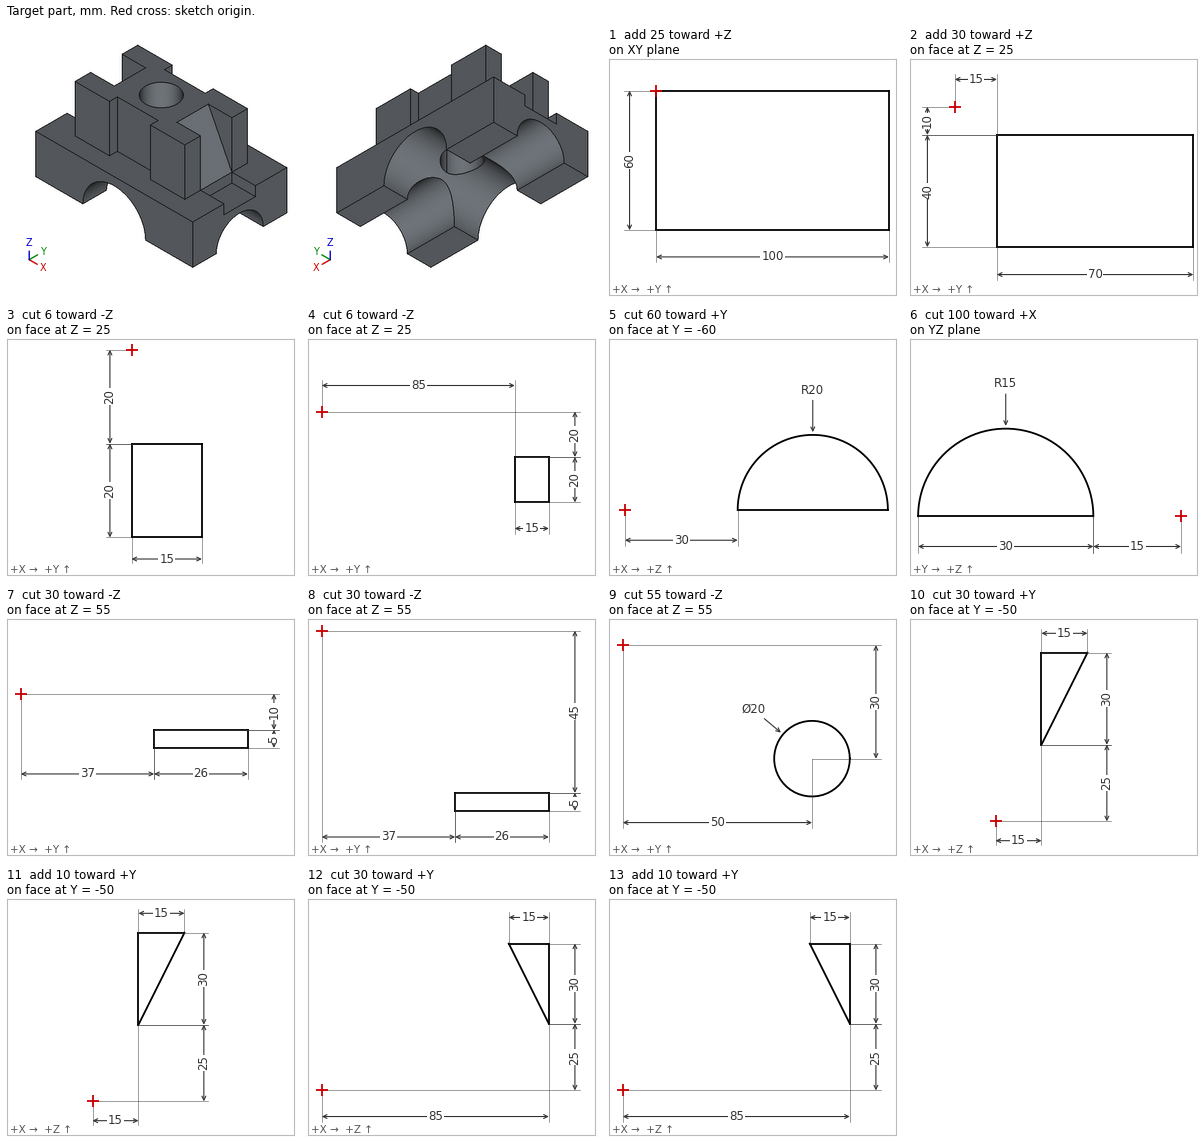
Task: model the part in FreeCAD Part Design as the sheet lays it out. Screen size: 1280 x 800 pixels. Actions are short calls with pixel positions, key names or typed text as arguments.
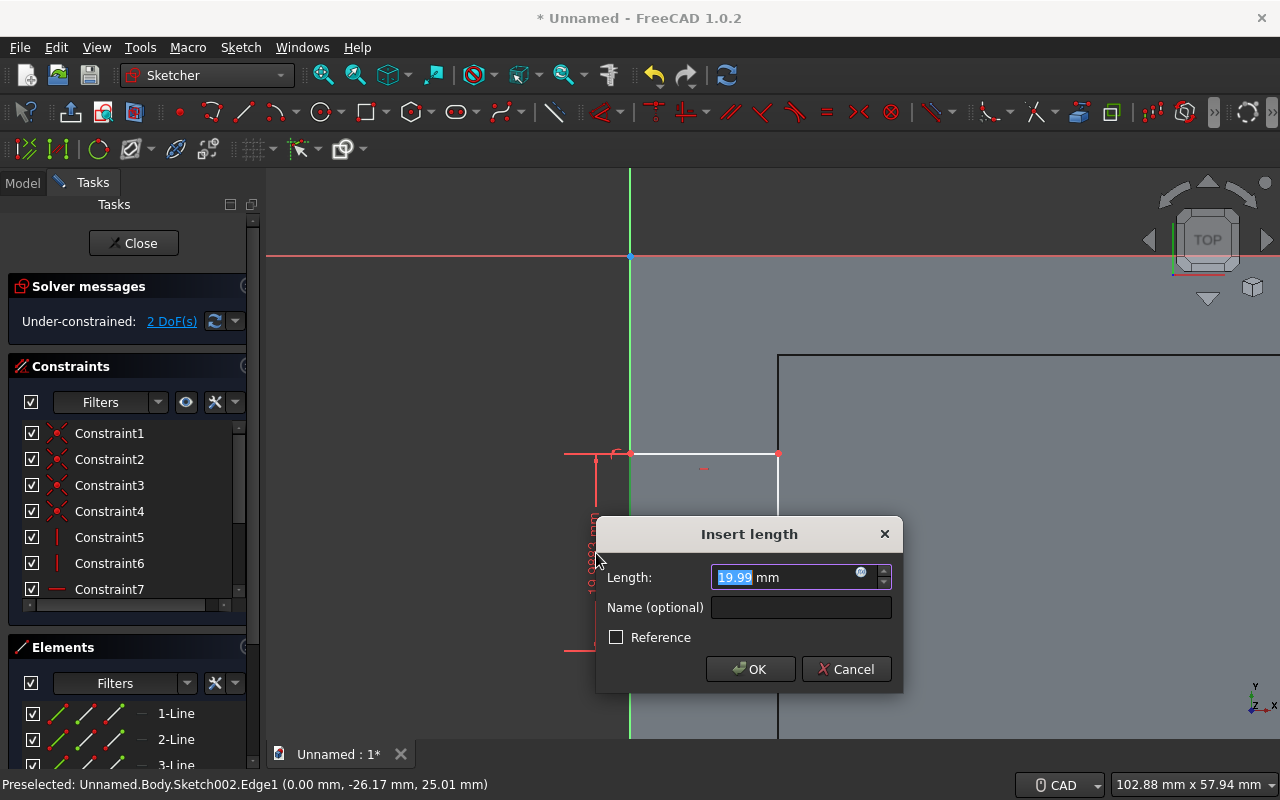
text(20)
key(Return)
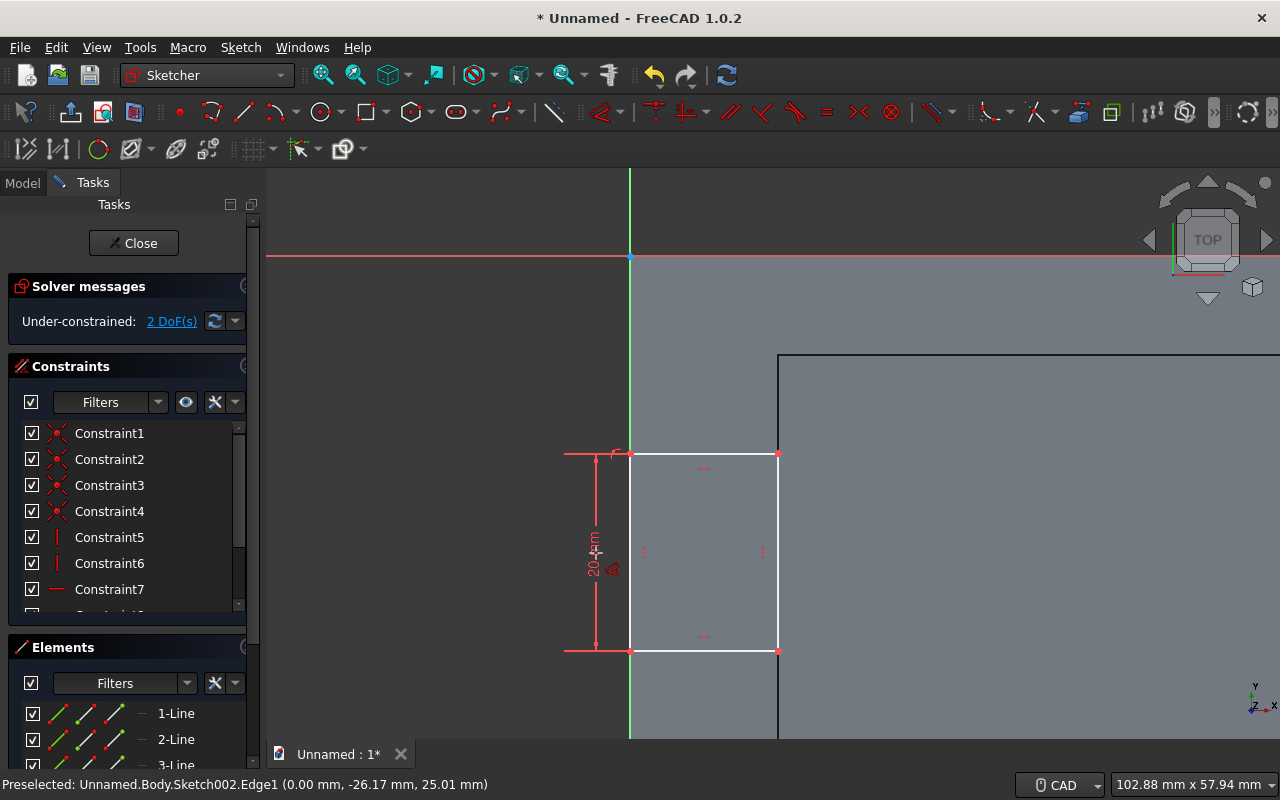
click(675, 651)
click(704, 685)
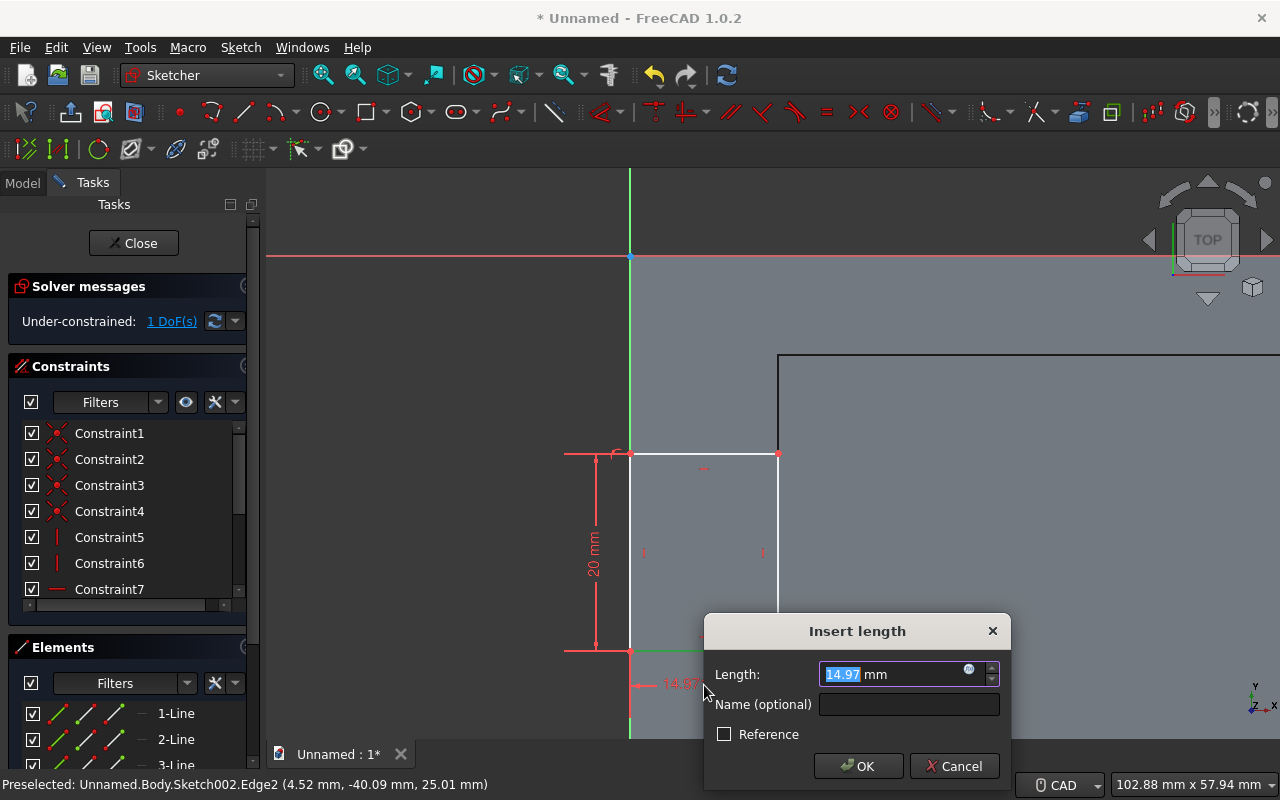
text(15)
key(Return)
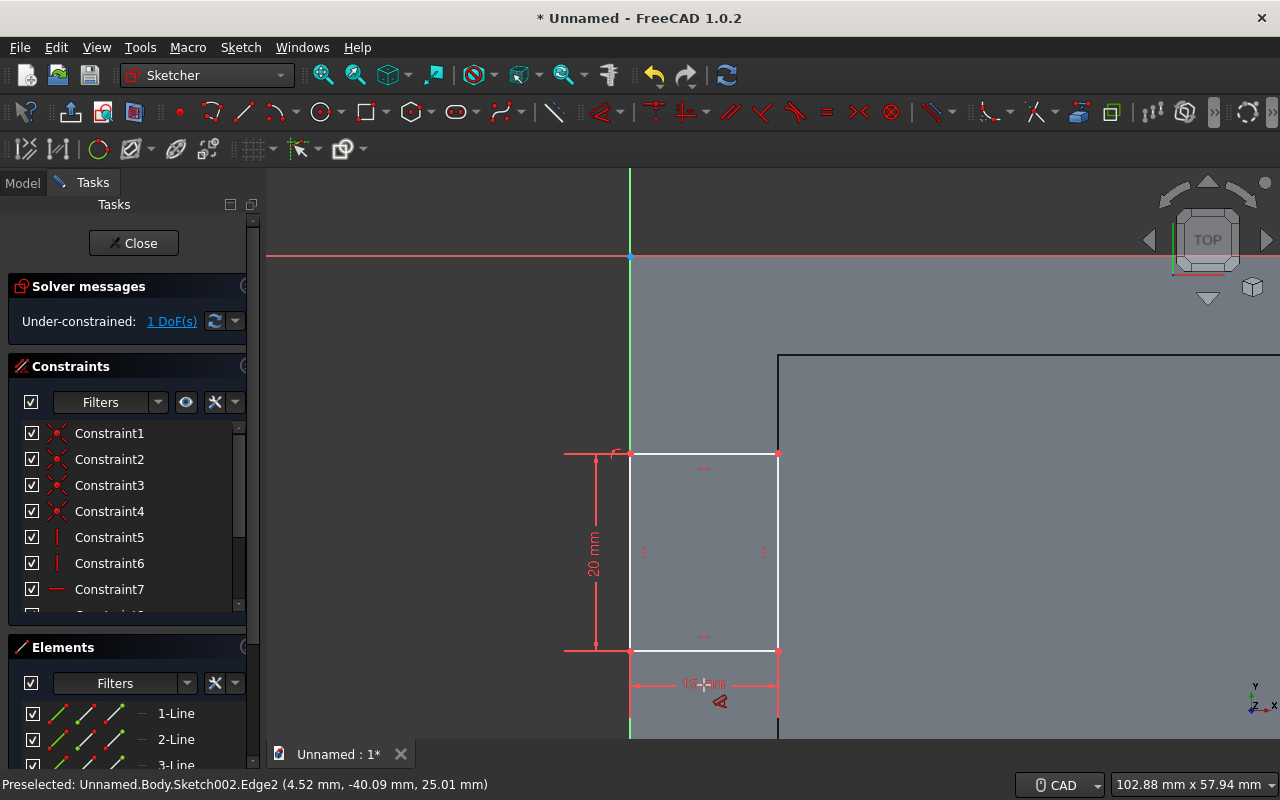
click(630, 454)
click(596, 355)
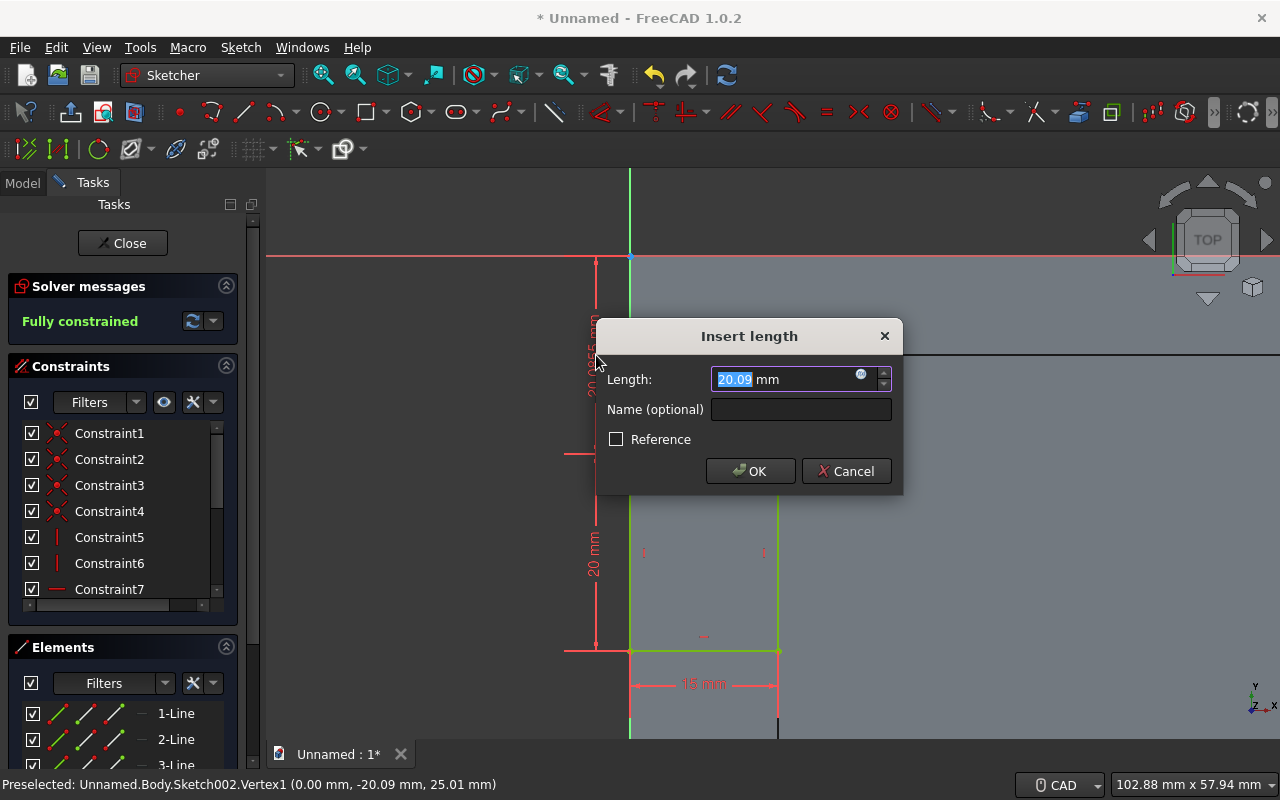
text(20)
key(Return)
key(Escape)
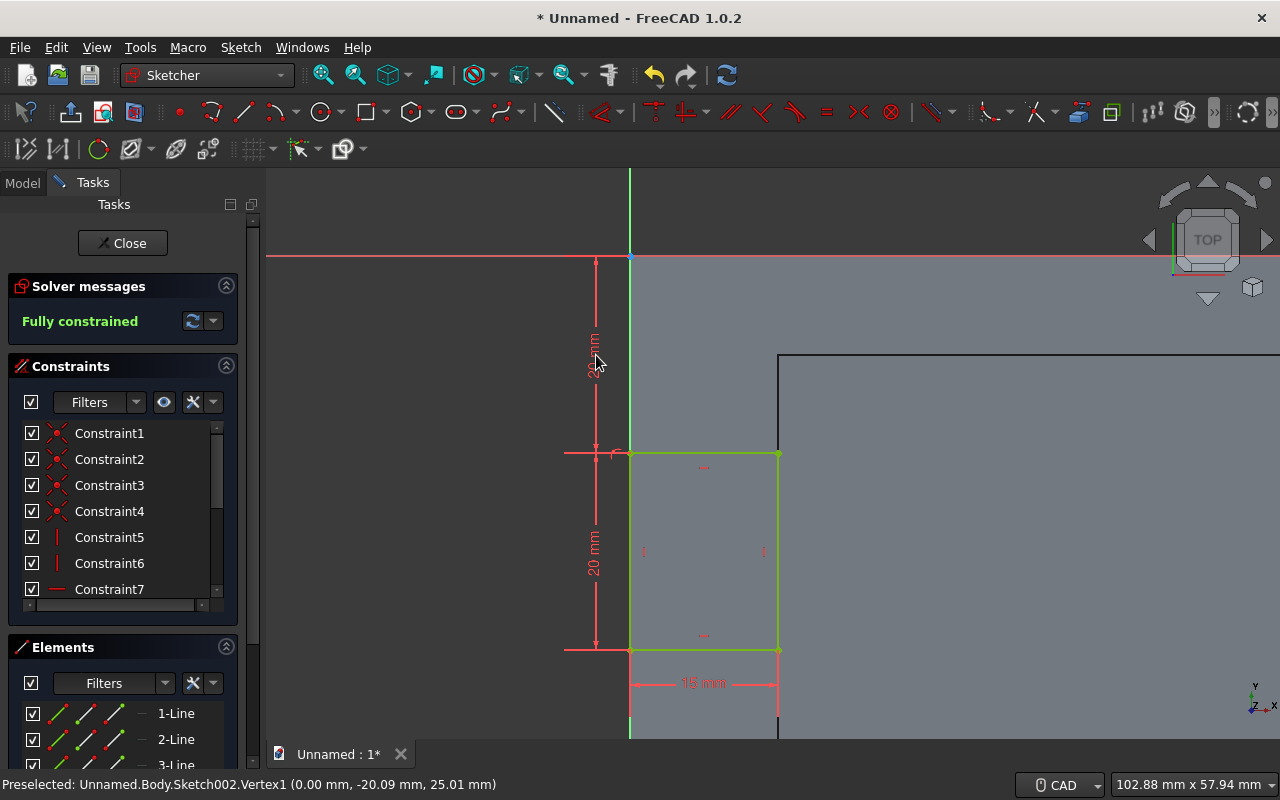
click(123, 243)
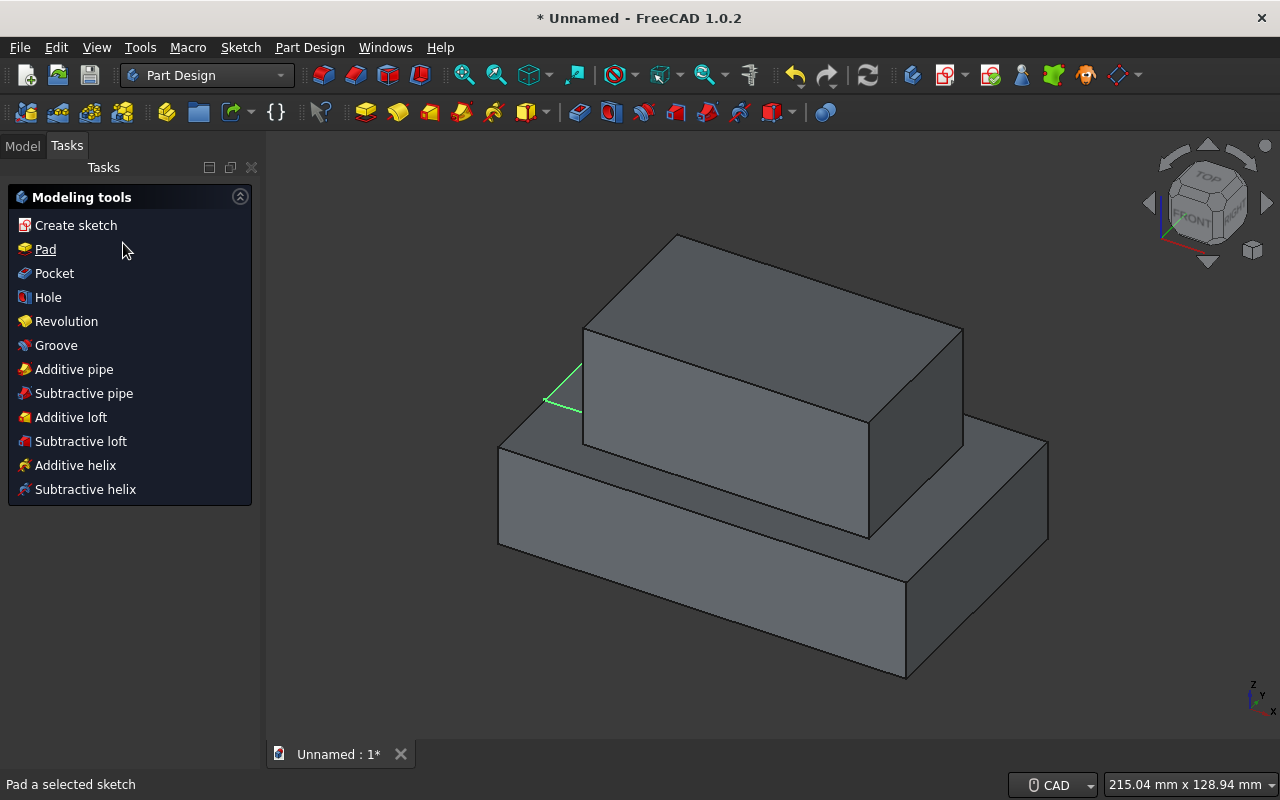
click(580, 112)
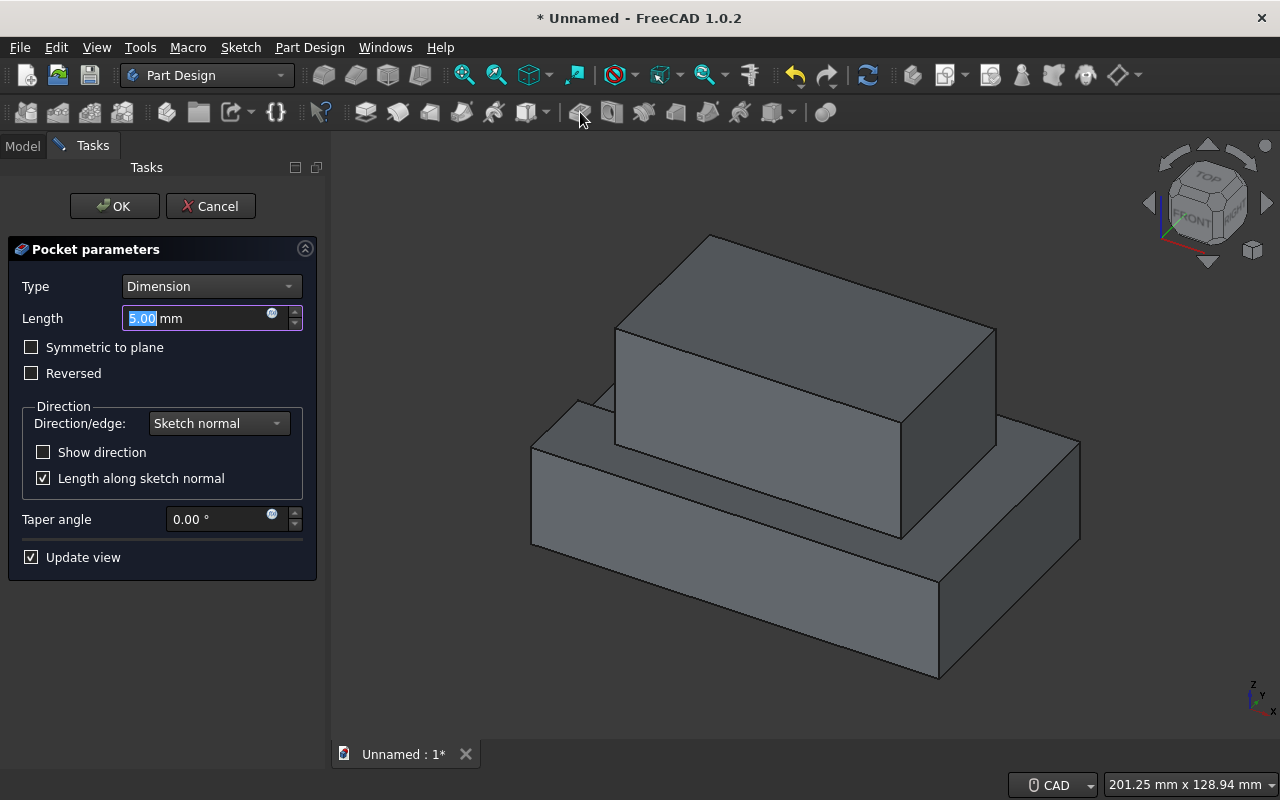
text(6)
key(Tab)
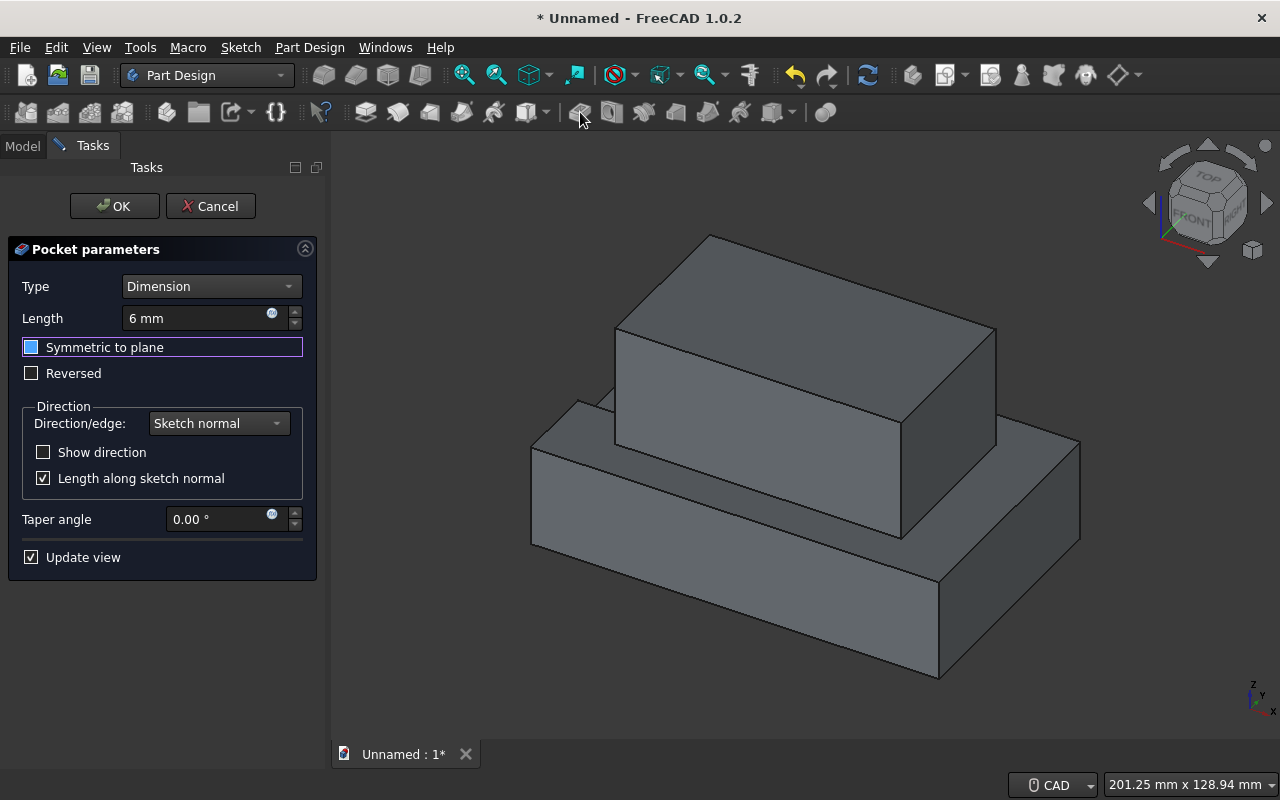
click(115, 206)